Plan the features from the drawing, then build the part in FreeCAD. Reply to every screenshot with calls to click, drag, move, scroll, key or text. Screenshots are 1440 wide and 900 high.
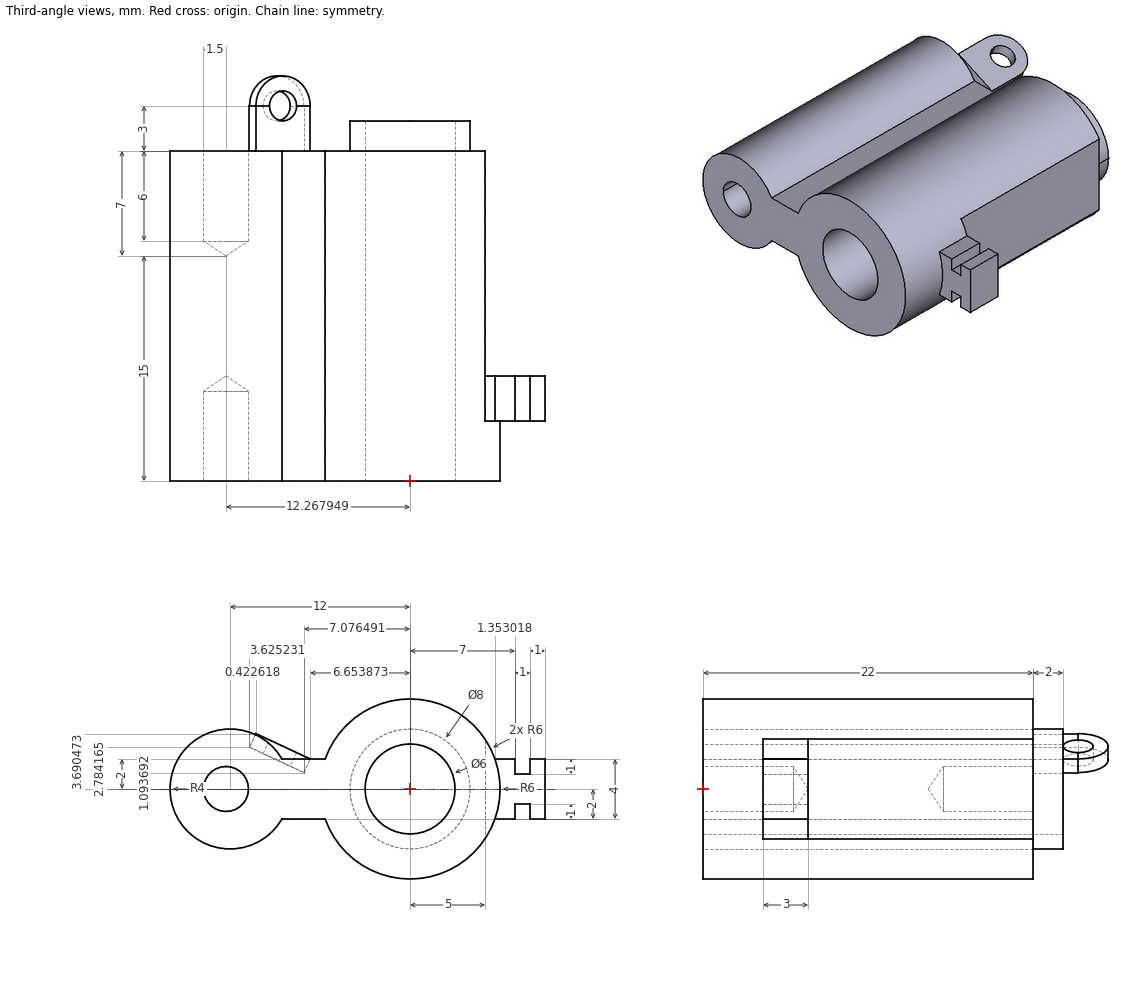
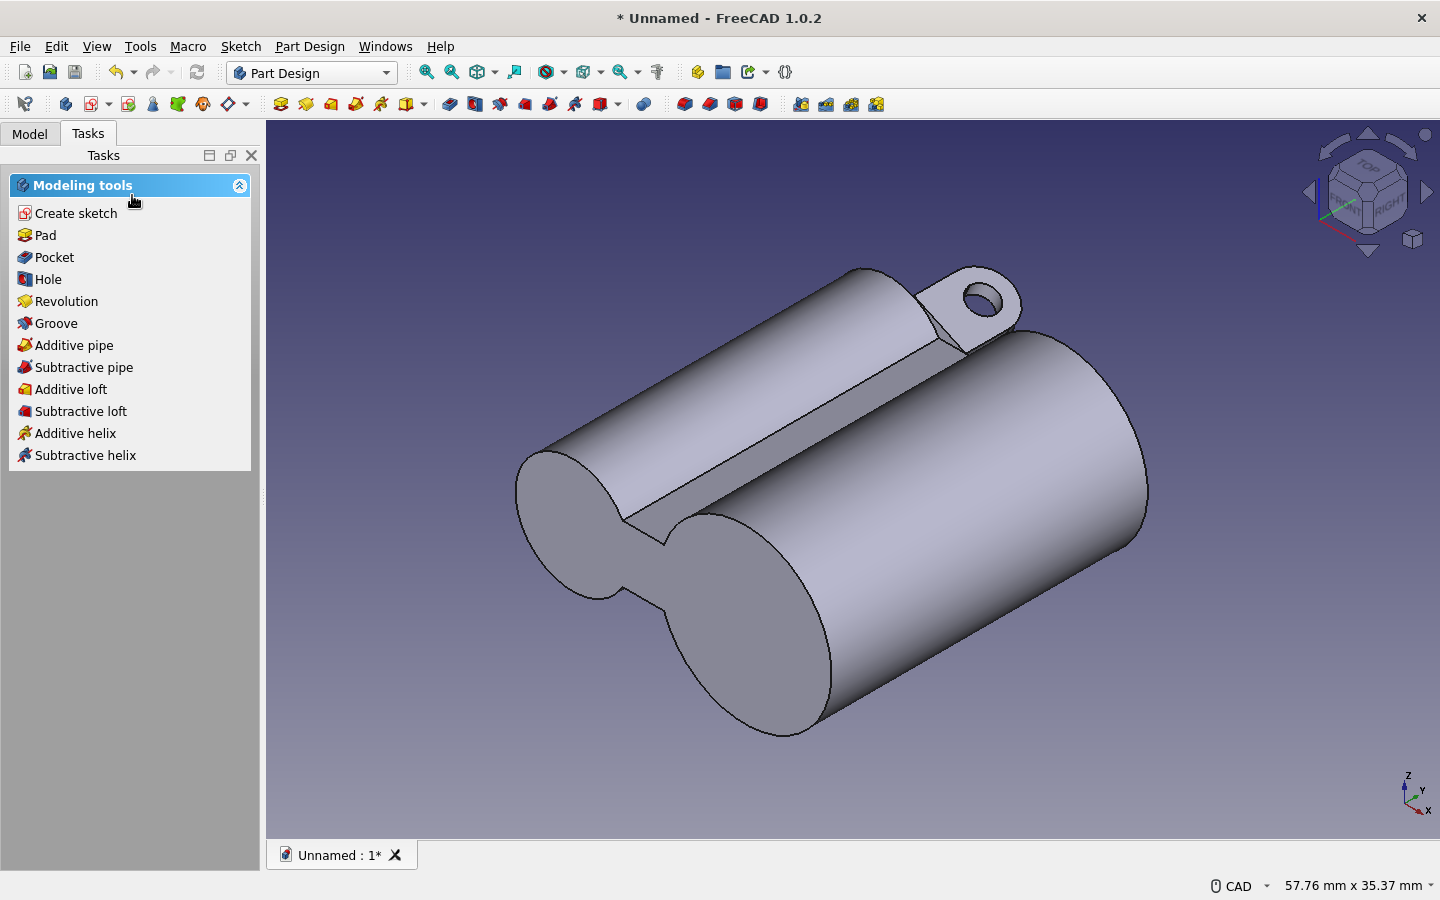
click(500, 104)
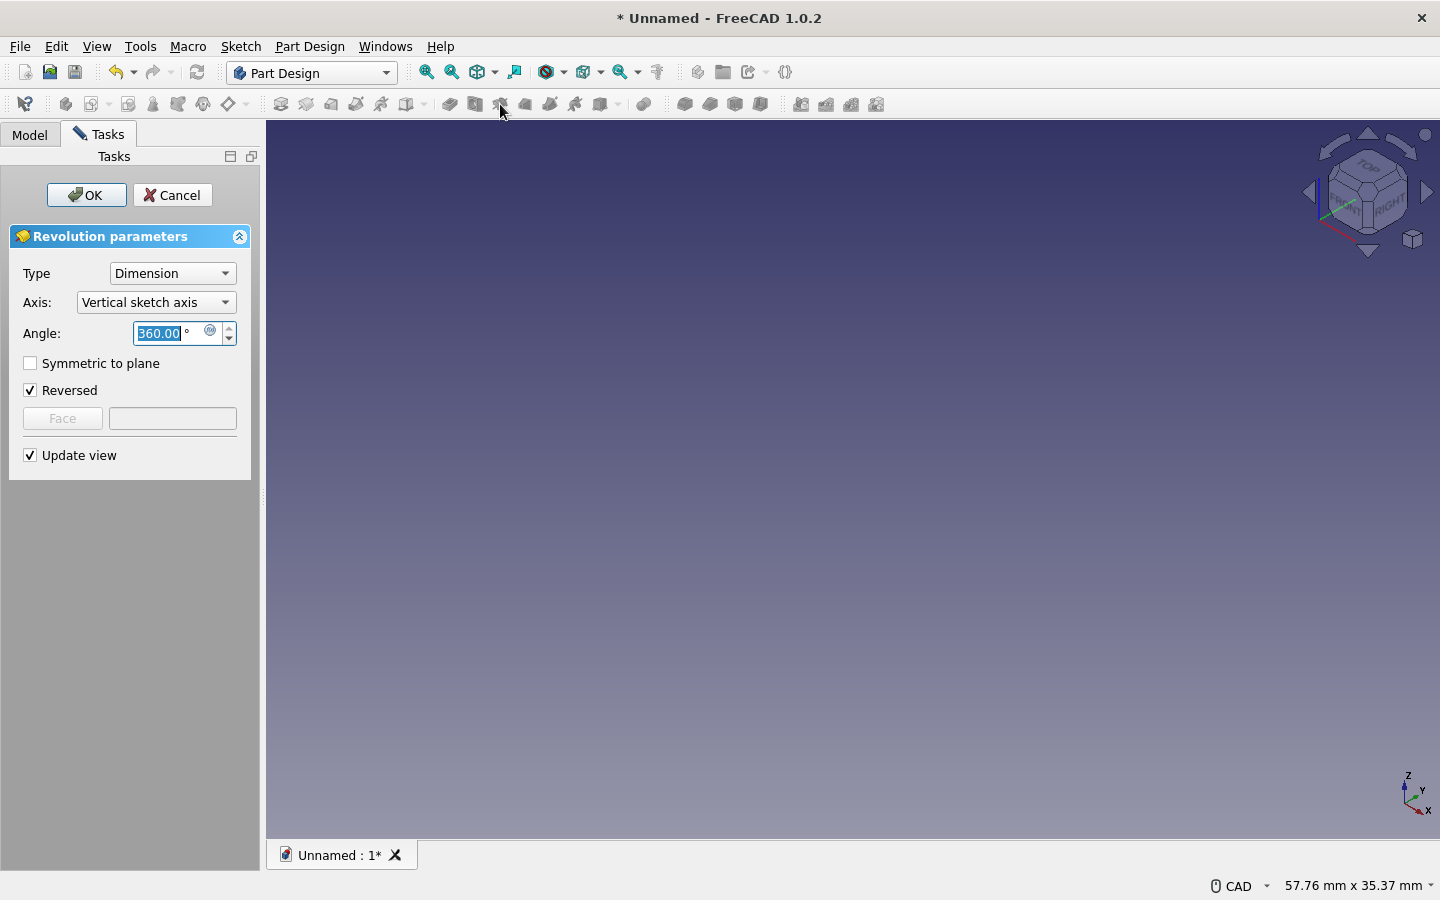
click(157, 302)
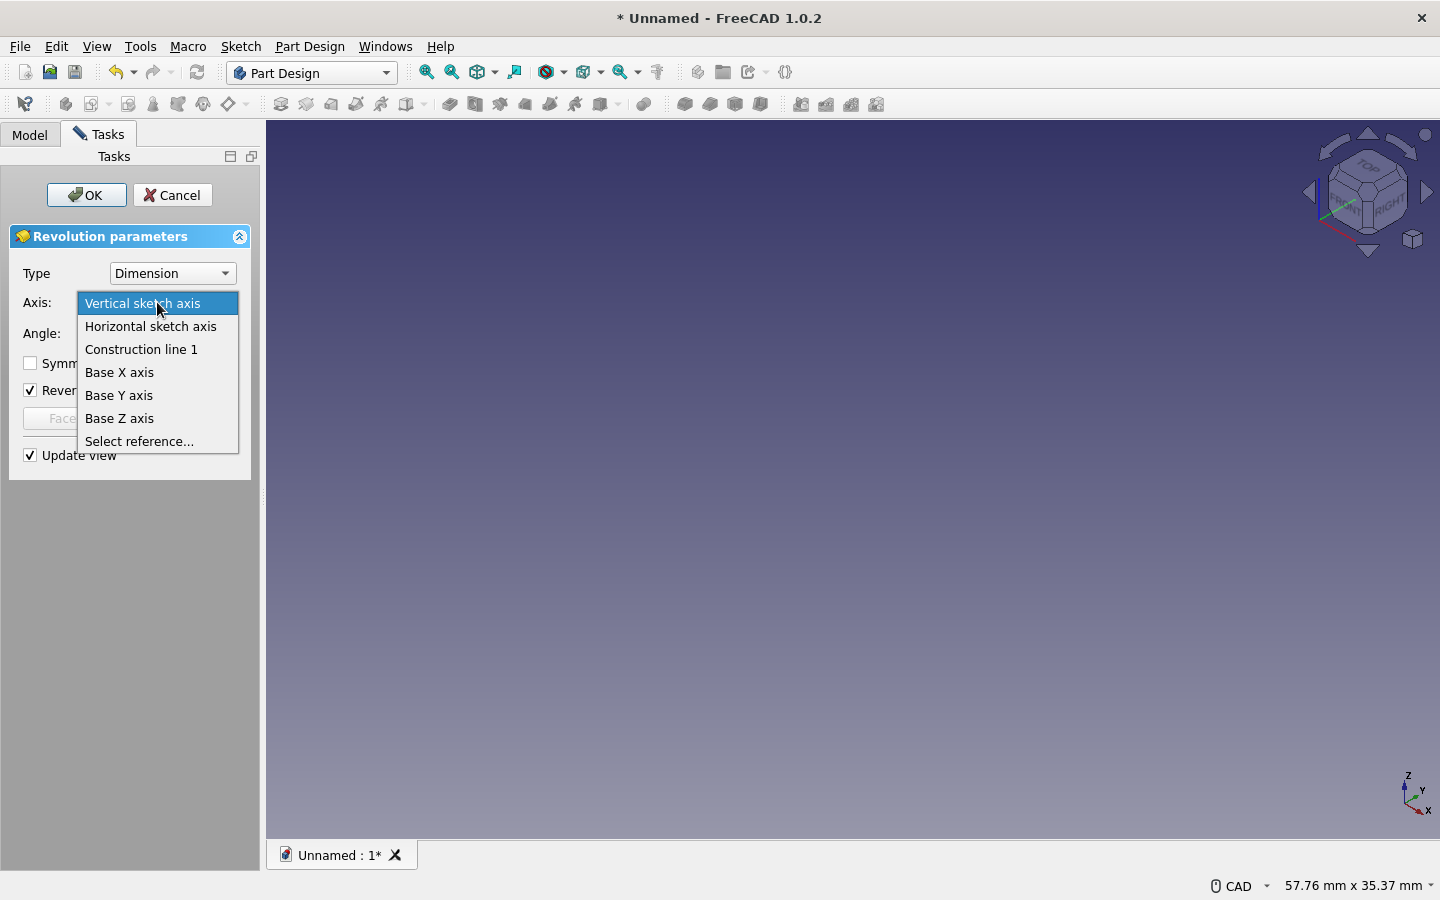
click(156, 350)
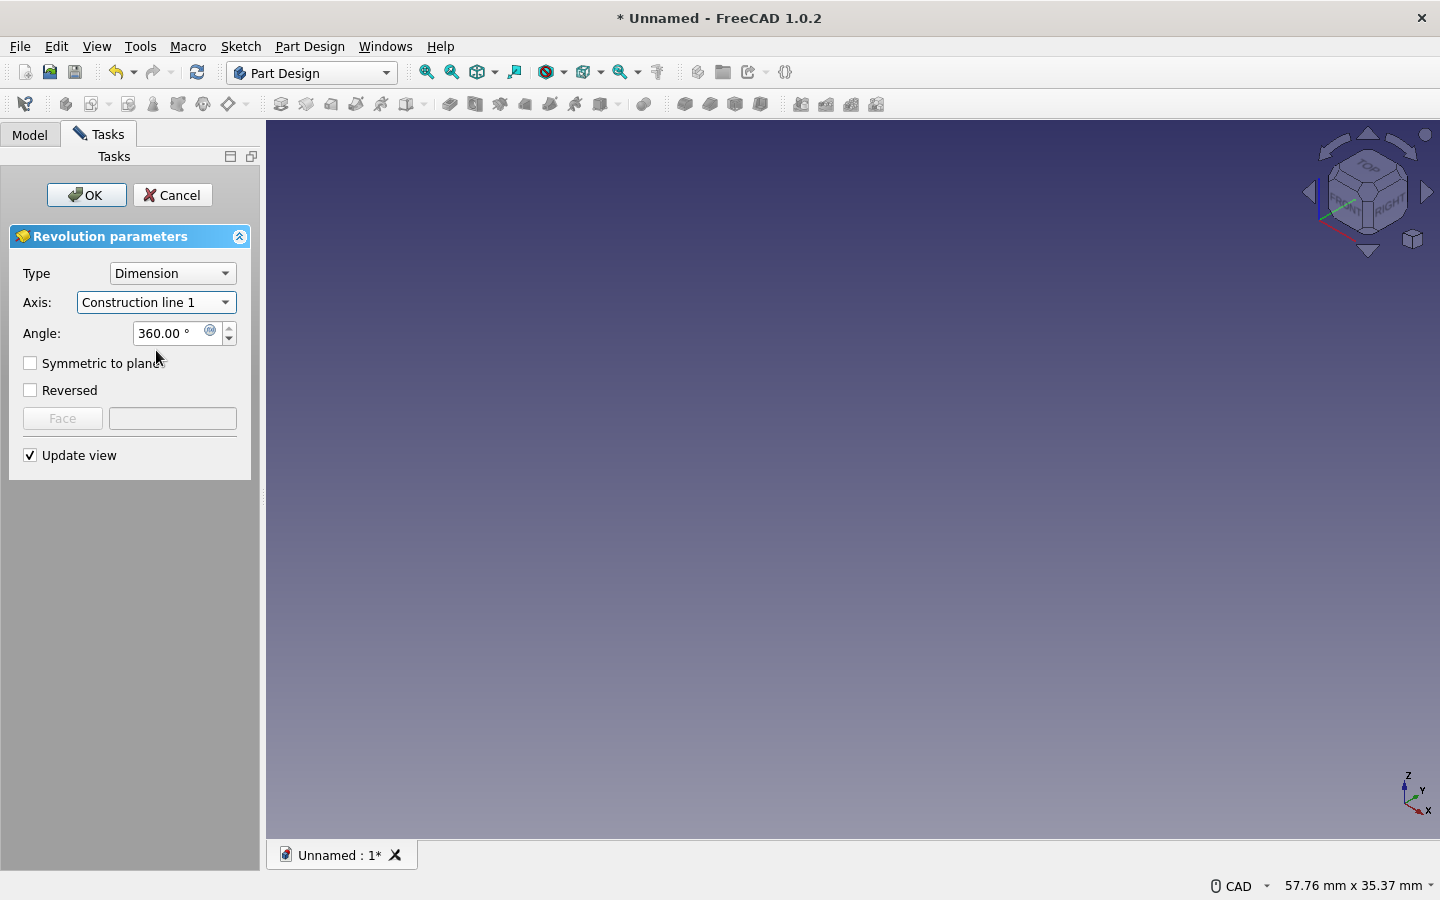
click(87, 195)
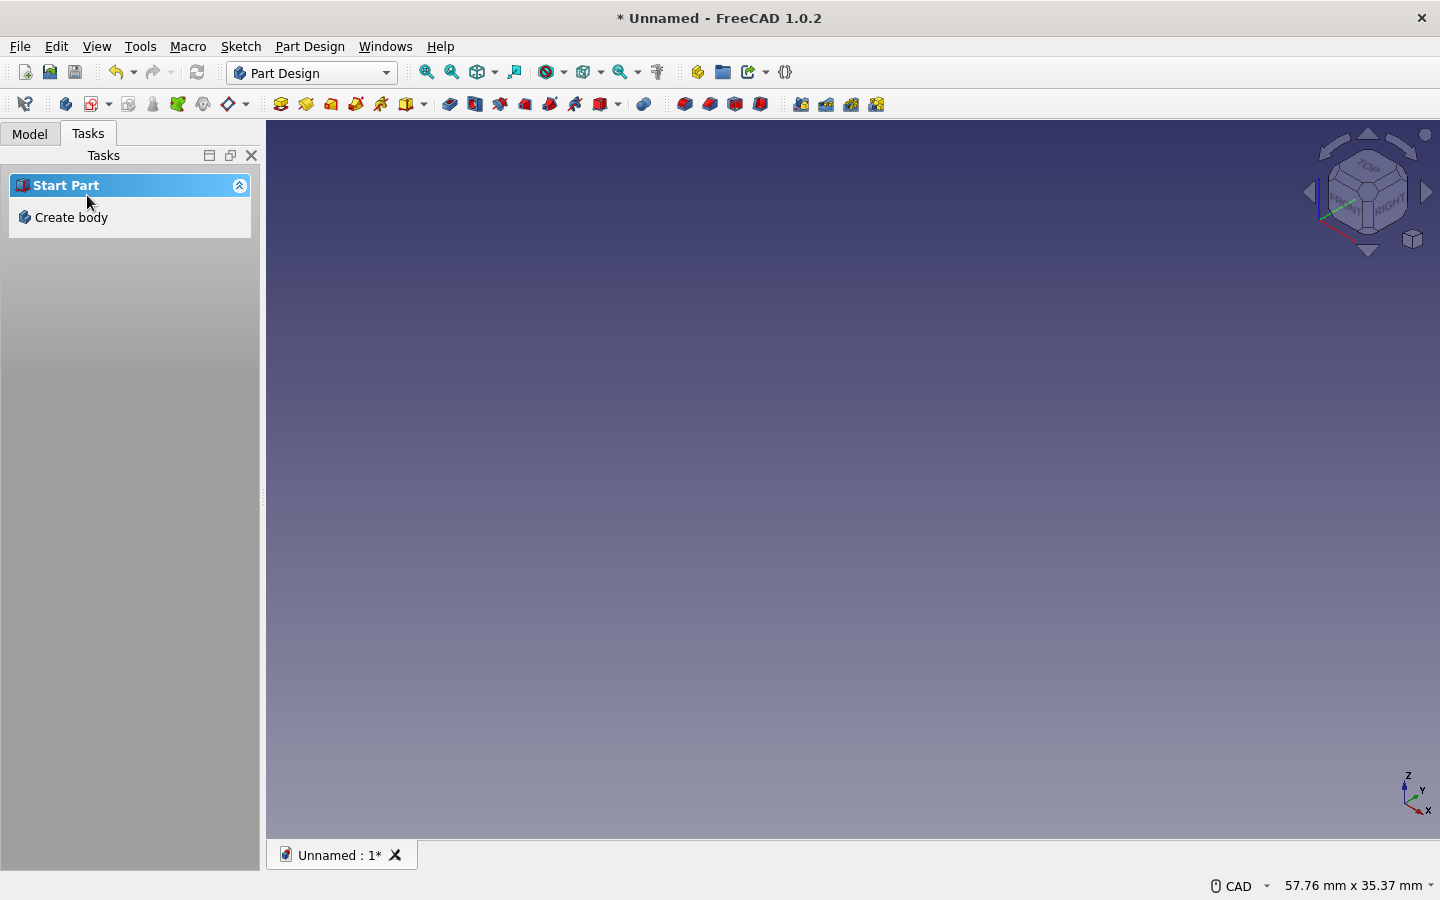
click(427, 72)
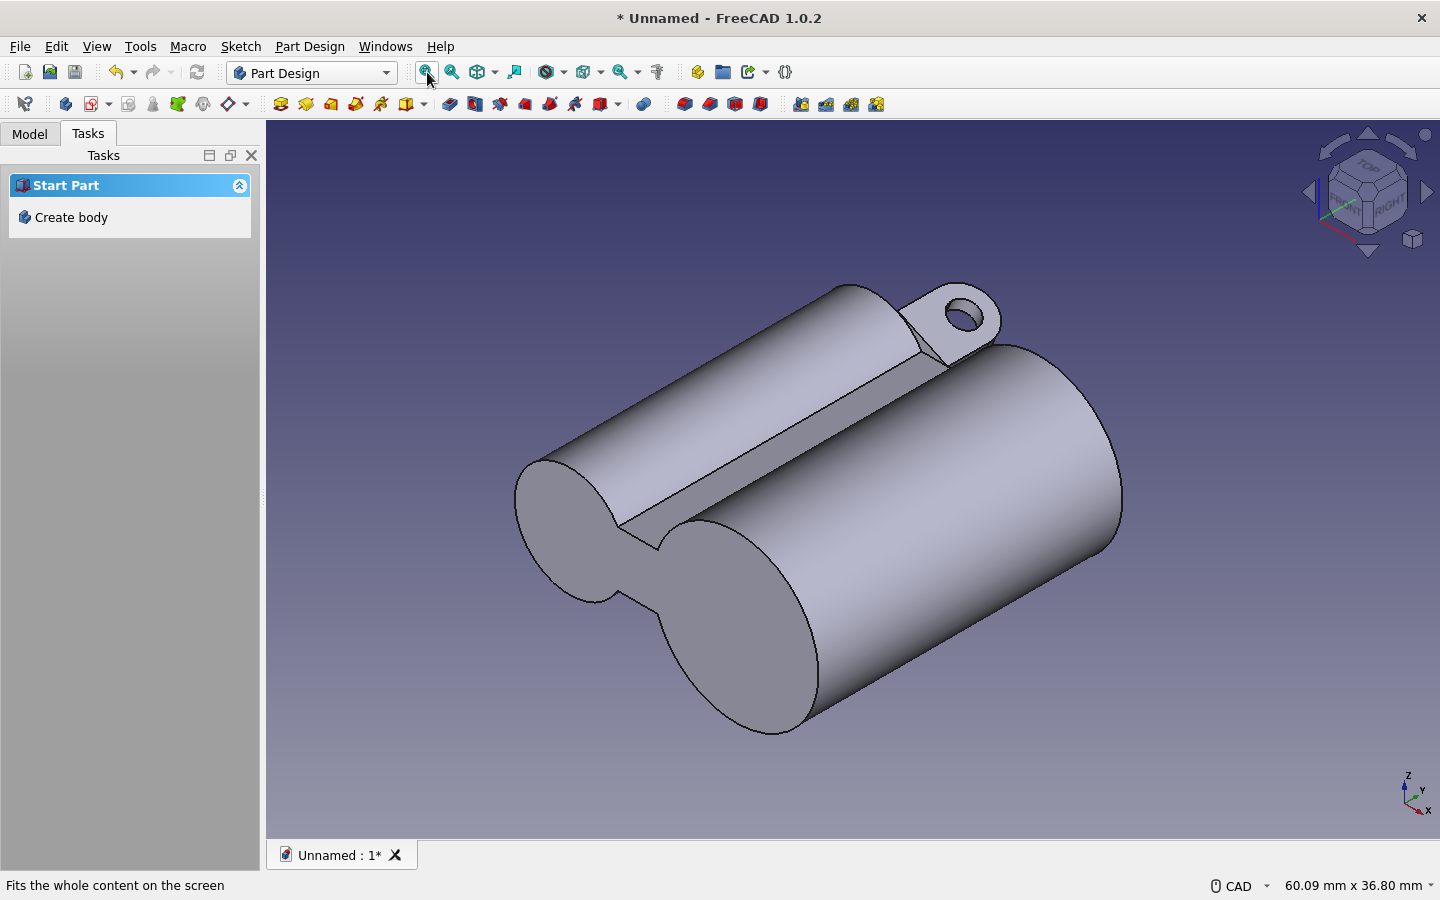
click(30, 134)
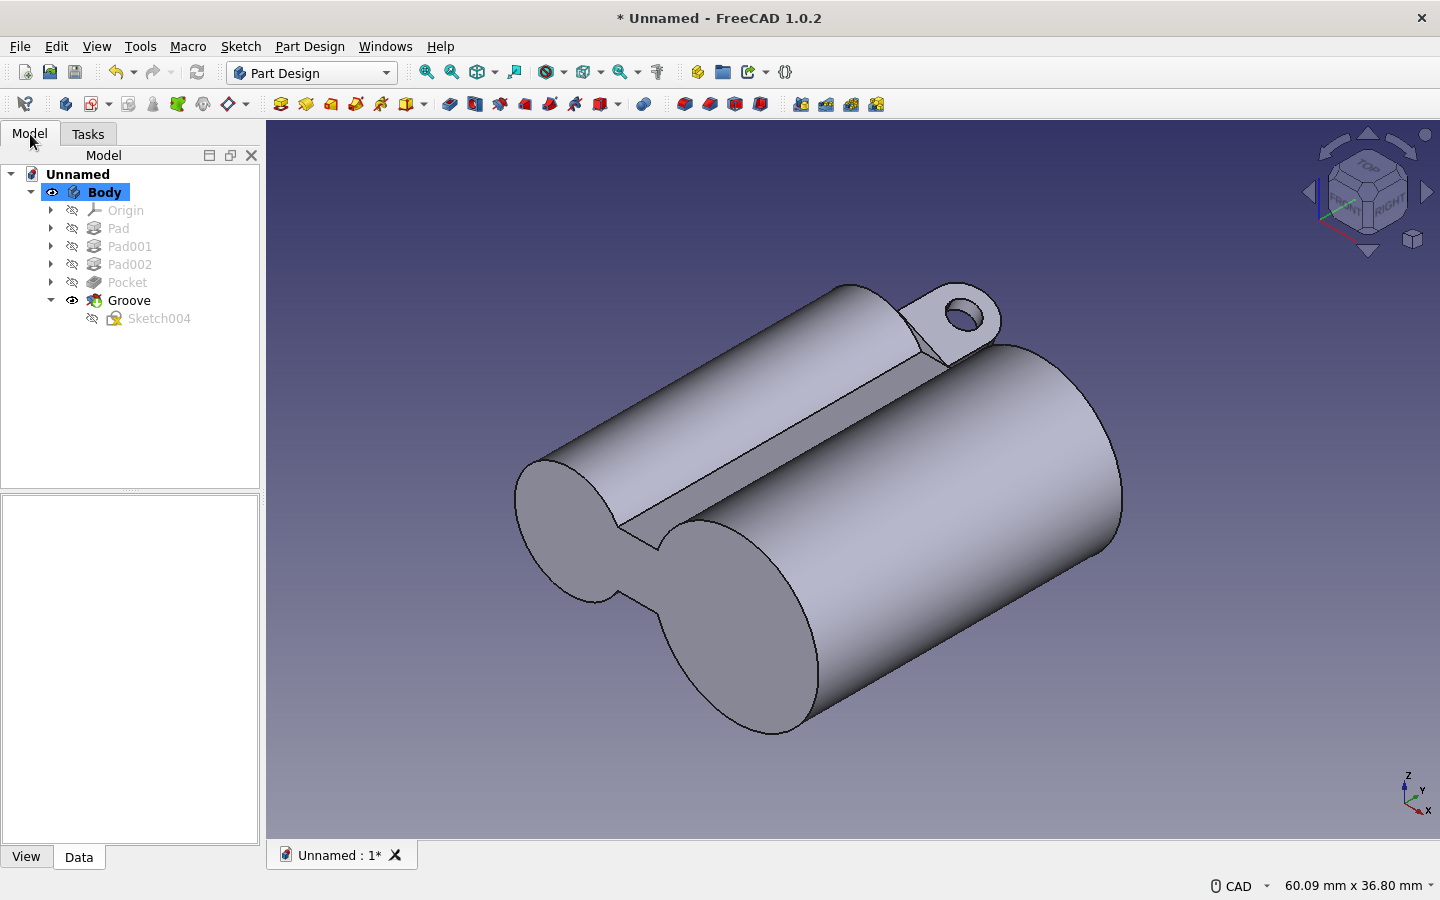
click(51, 210)